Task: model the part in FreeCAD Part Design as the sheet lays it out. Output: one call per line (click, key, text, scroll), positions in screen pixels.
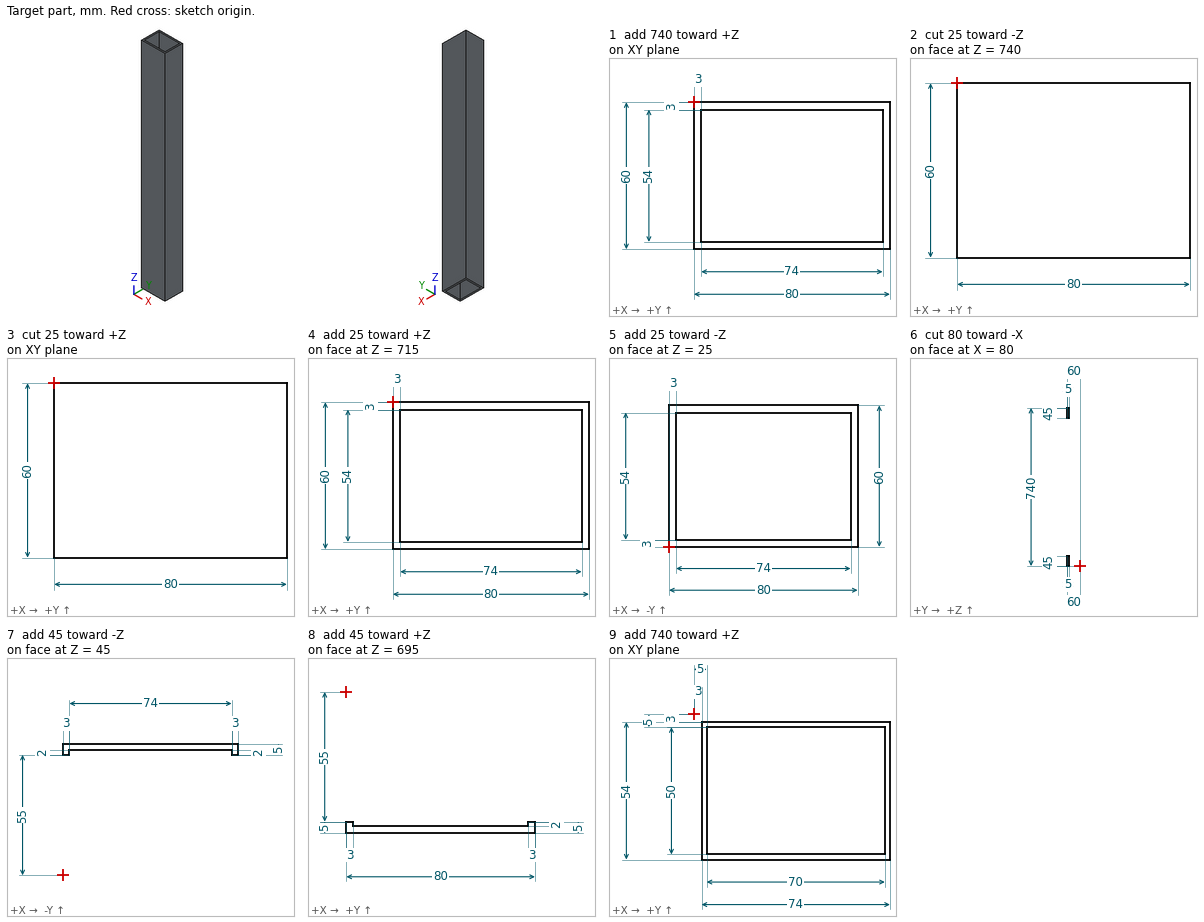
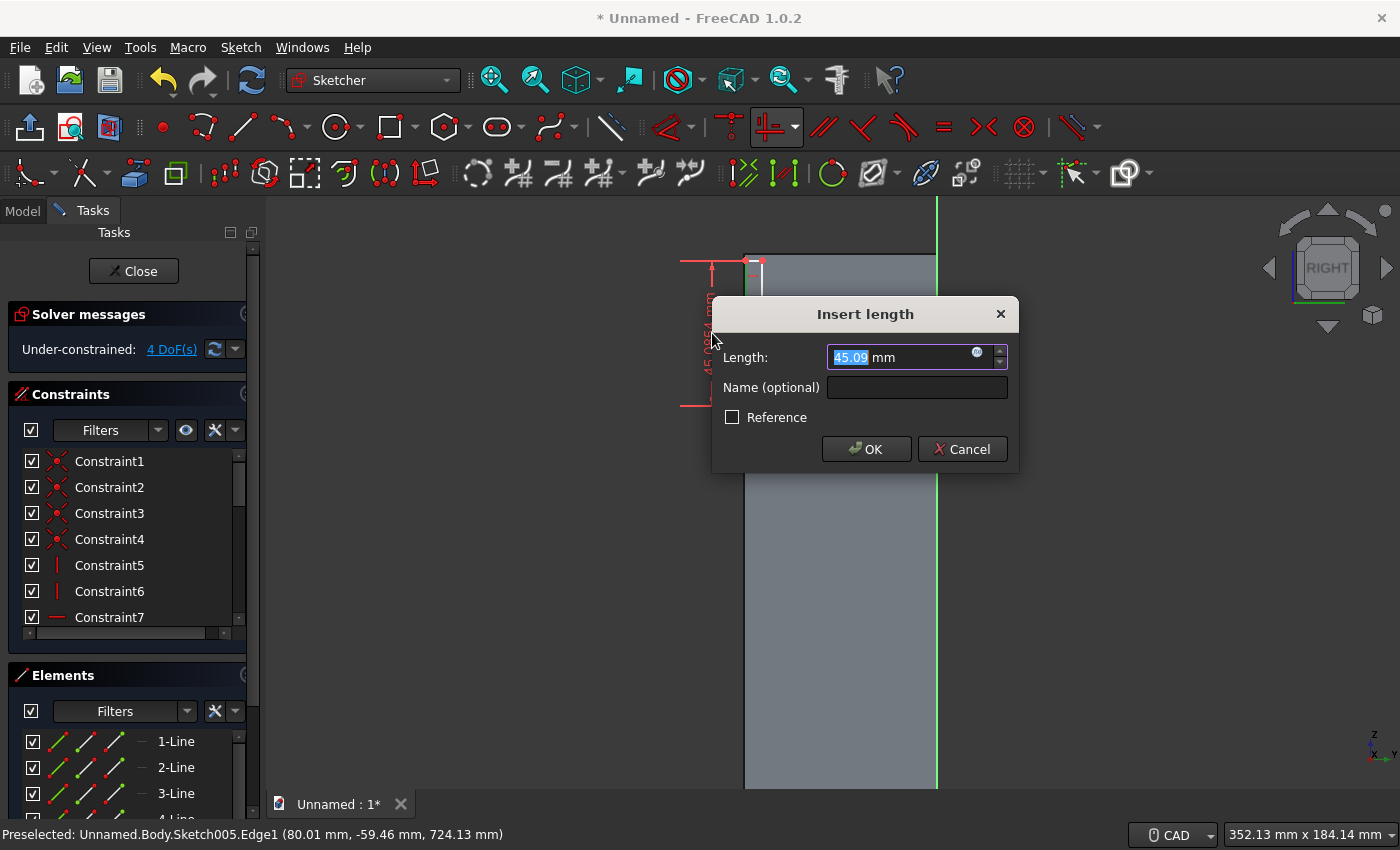
text(45)
key(Return)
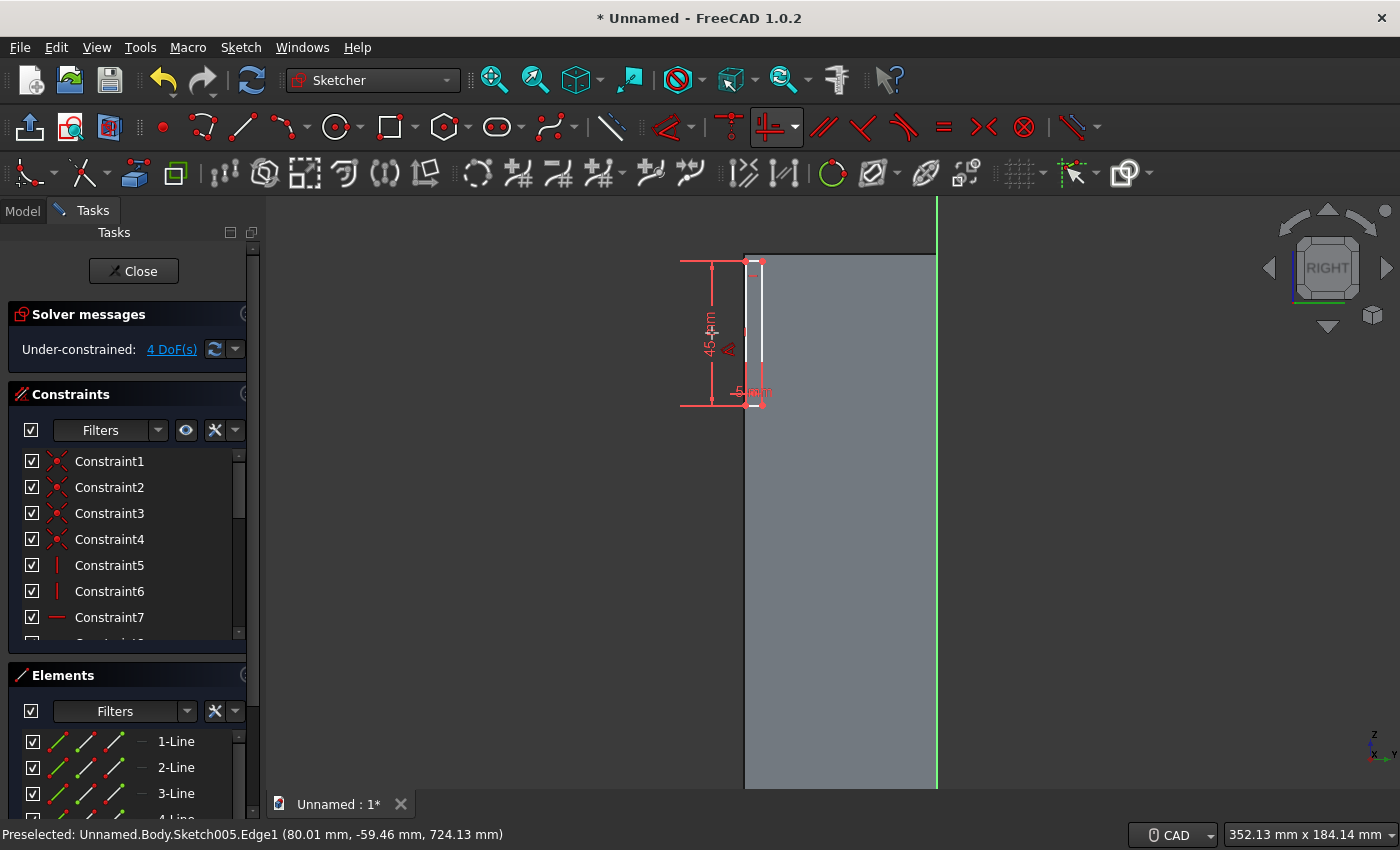
scroll(749, 304, down, 9)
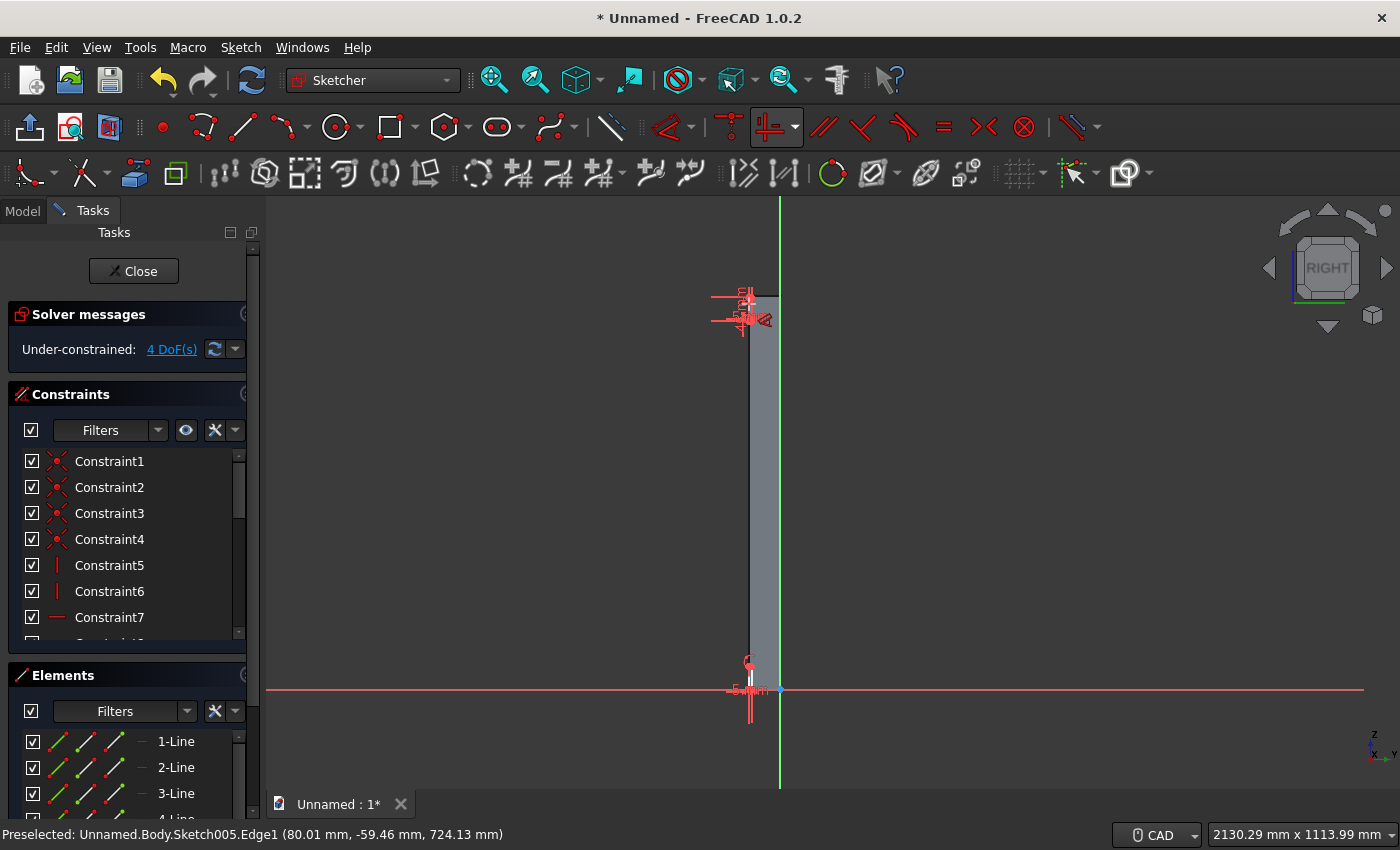
scroll(749, 674, up, 9)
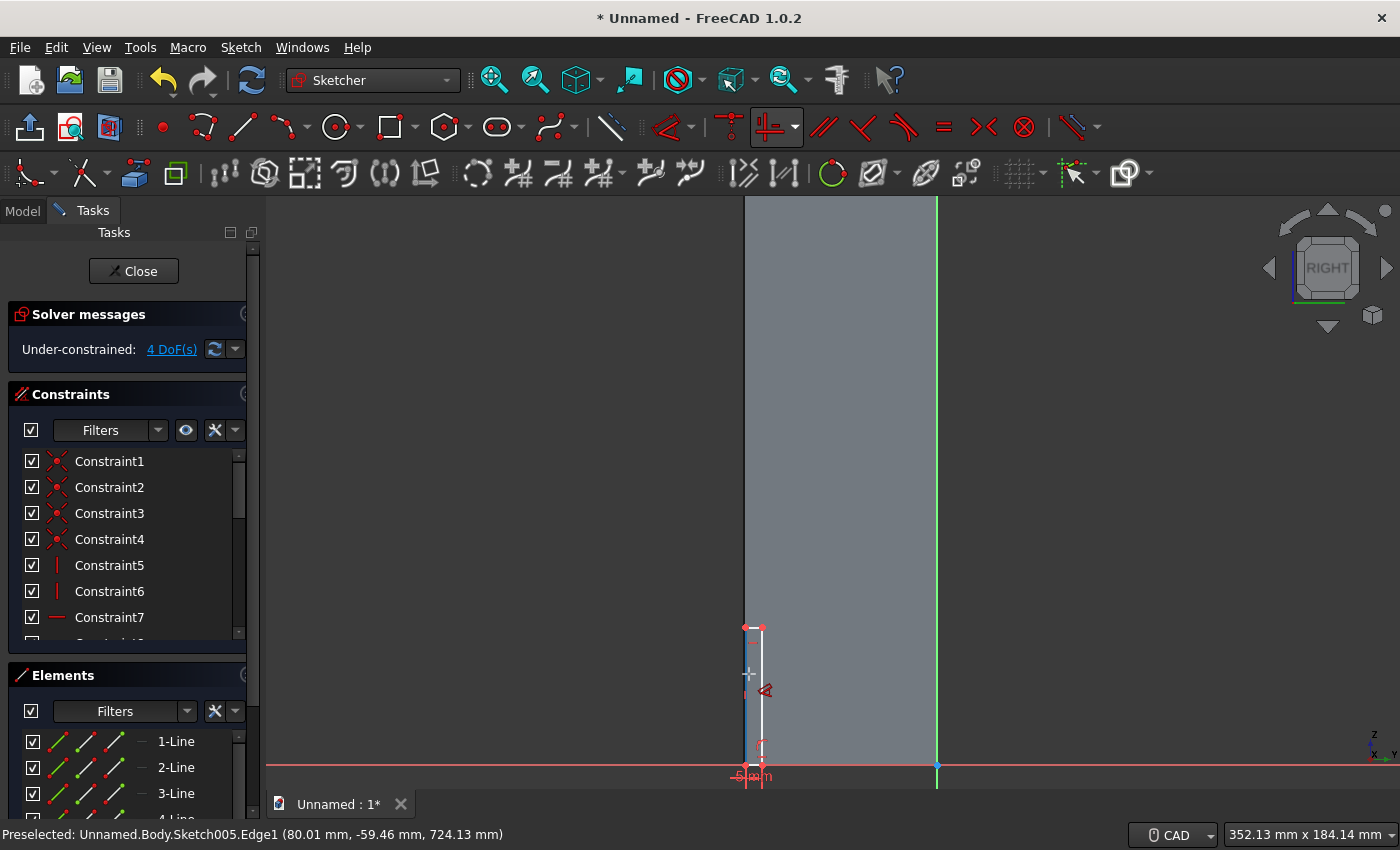
click(746, 669)
click(712, 694)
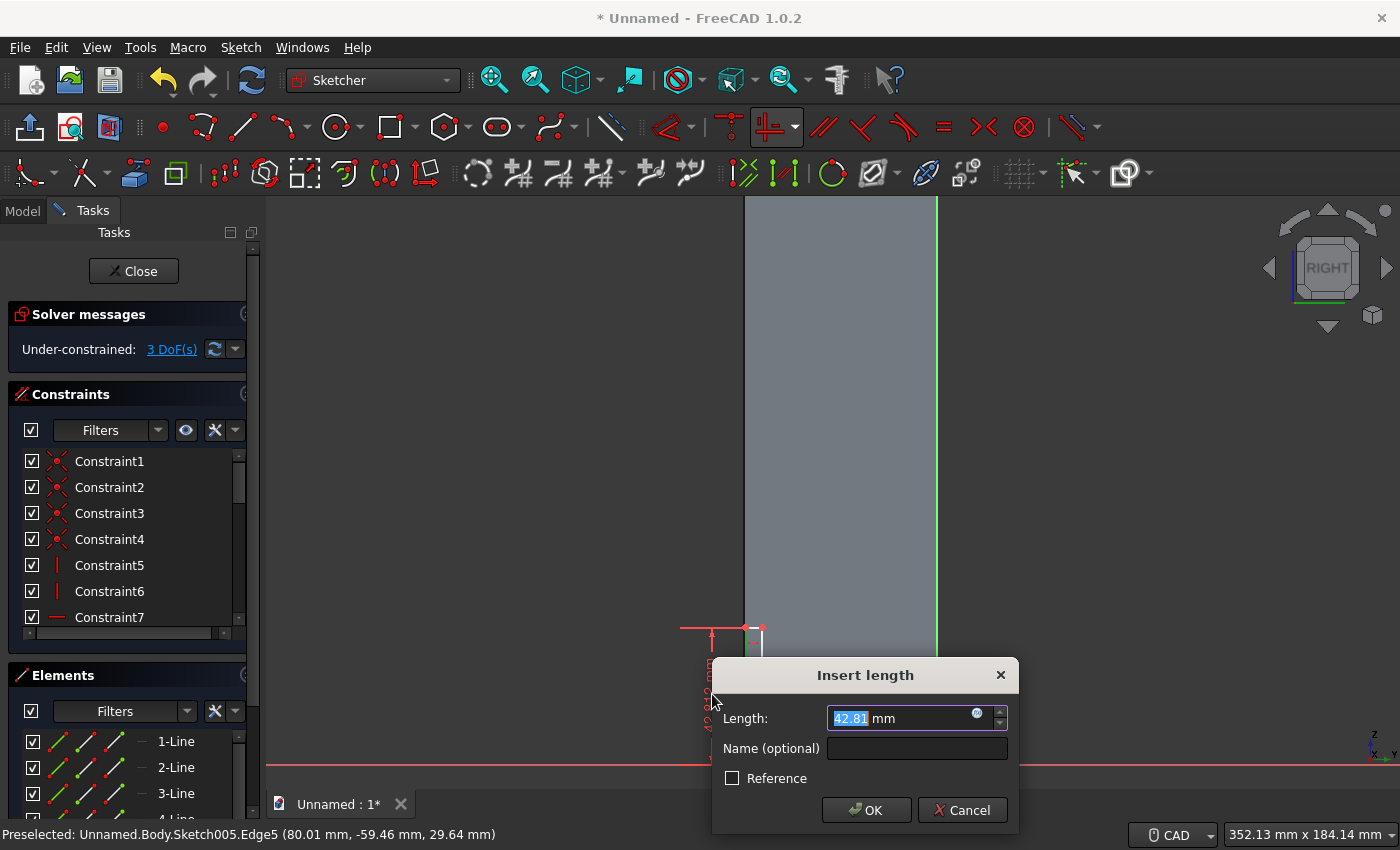
text(45)
key(Return)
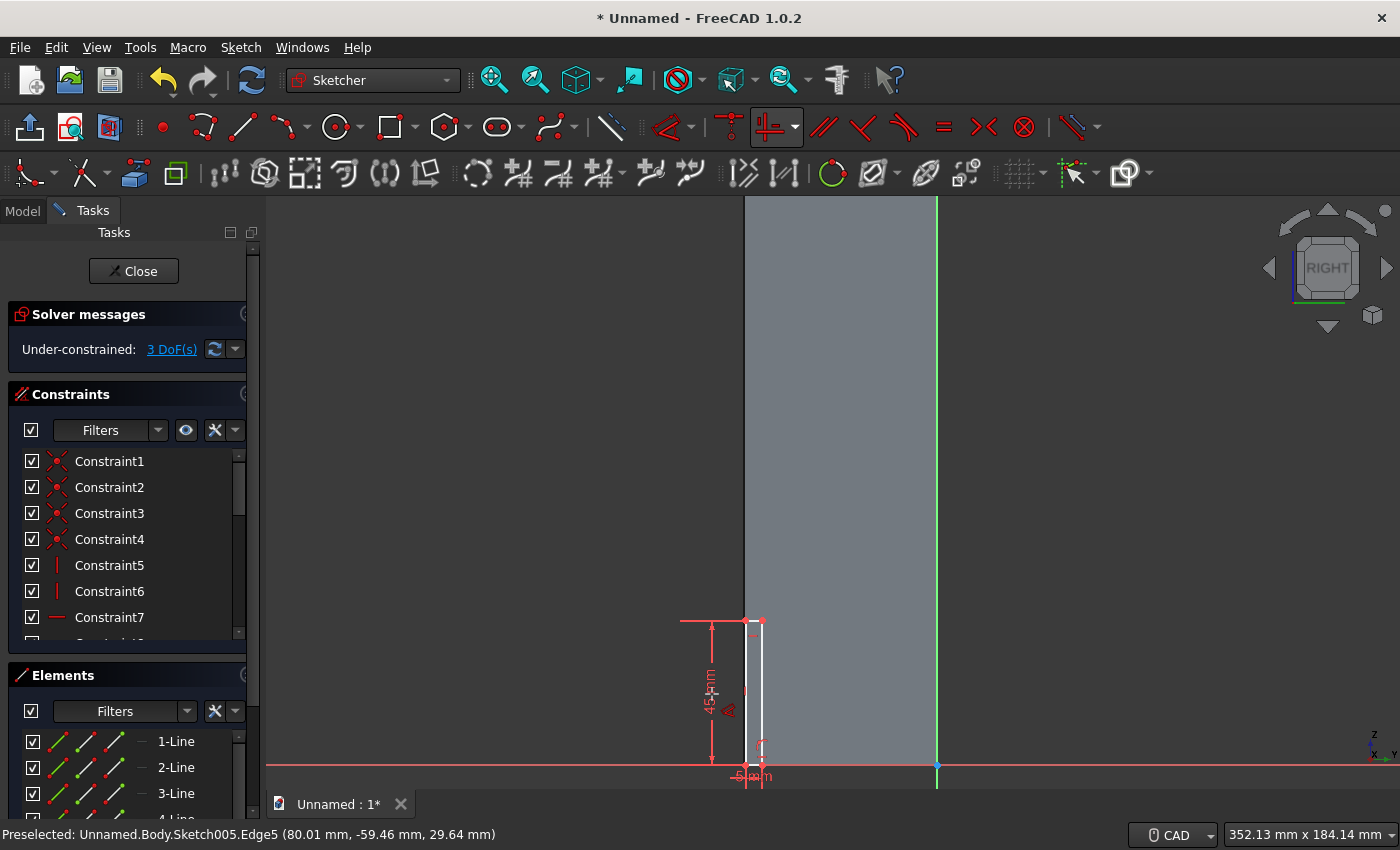
scroll(749, 674, down, 9)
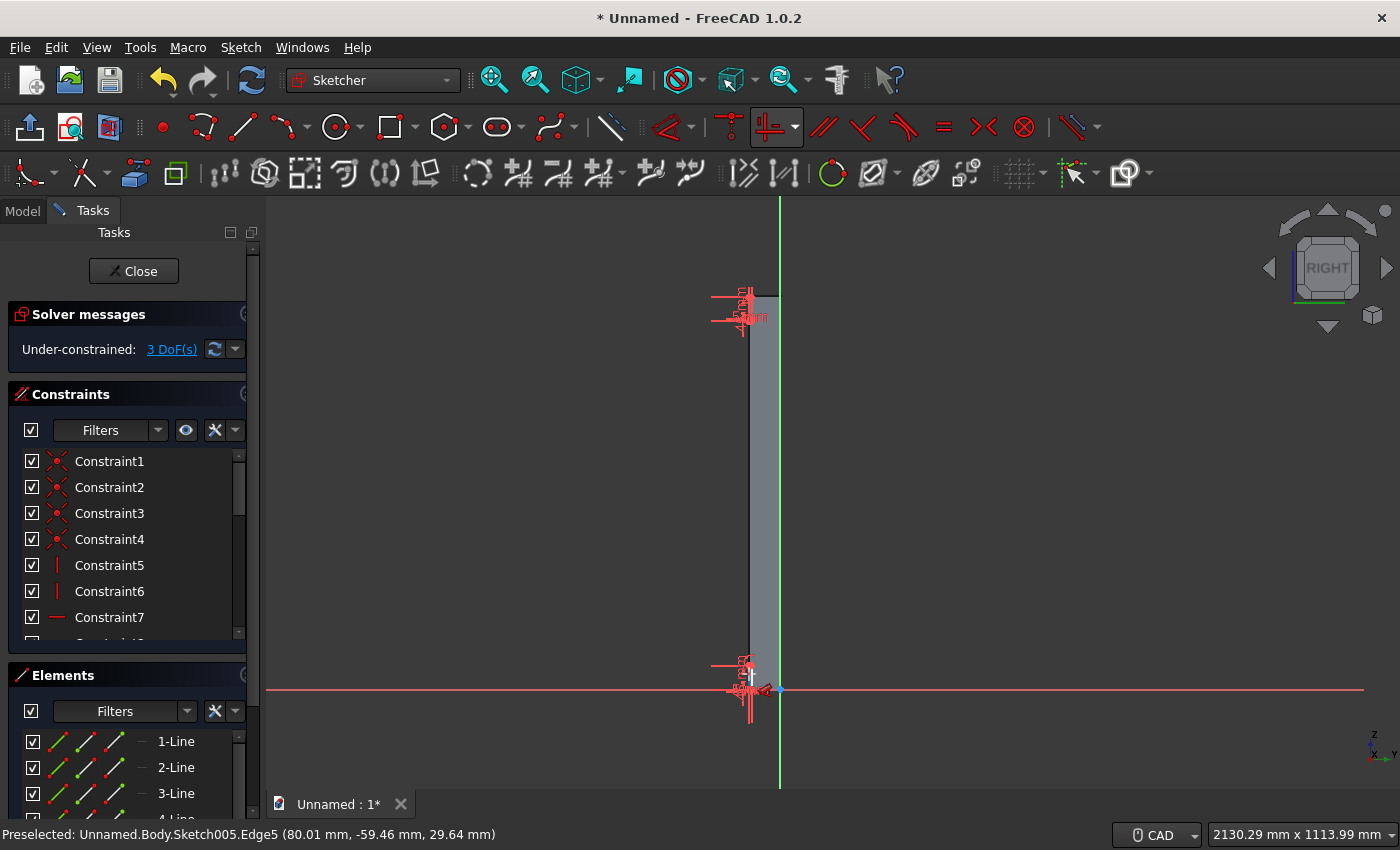
scroll(749, 297, up, 8)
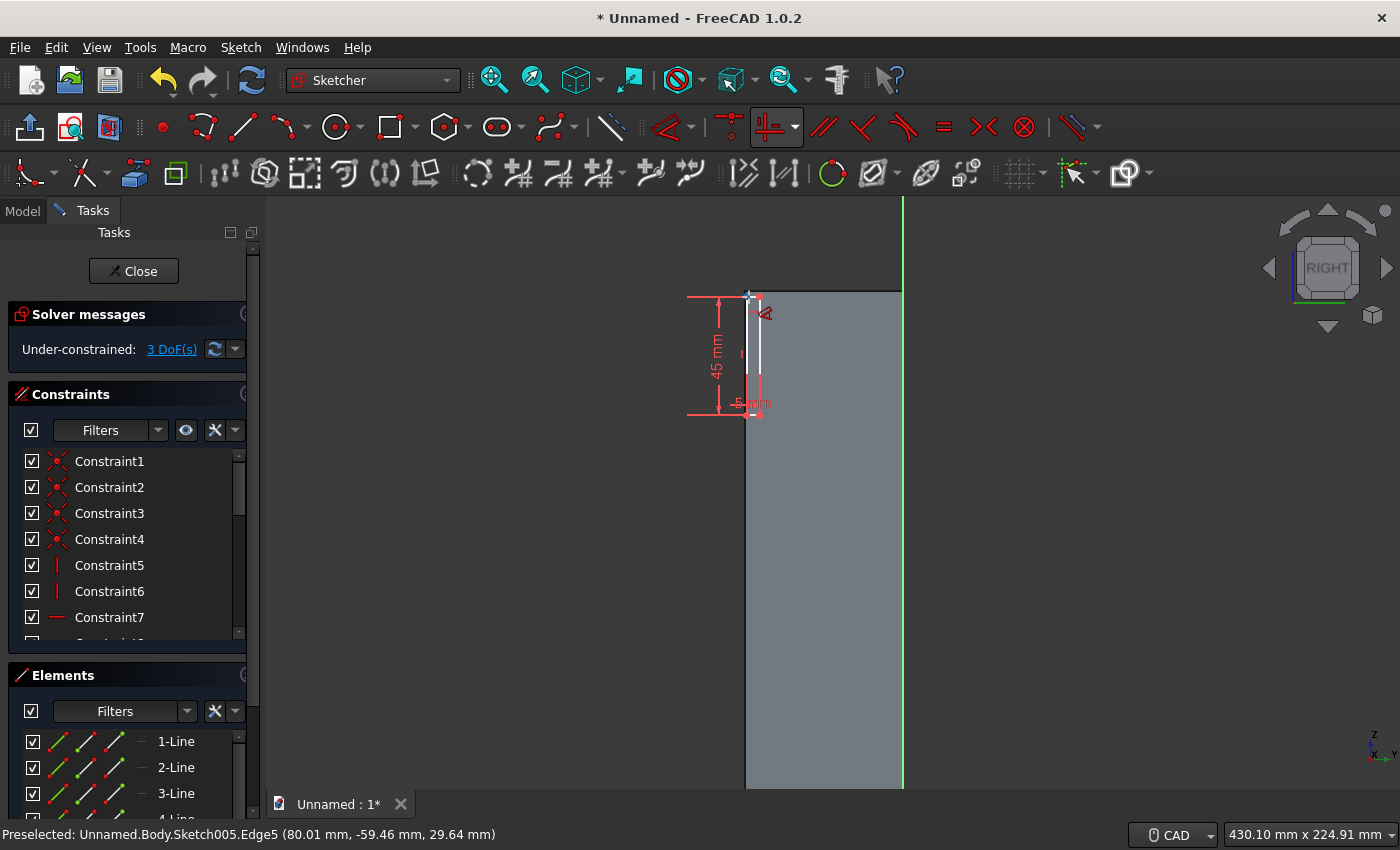
click(747, 297)
click(825, 263)